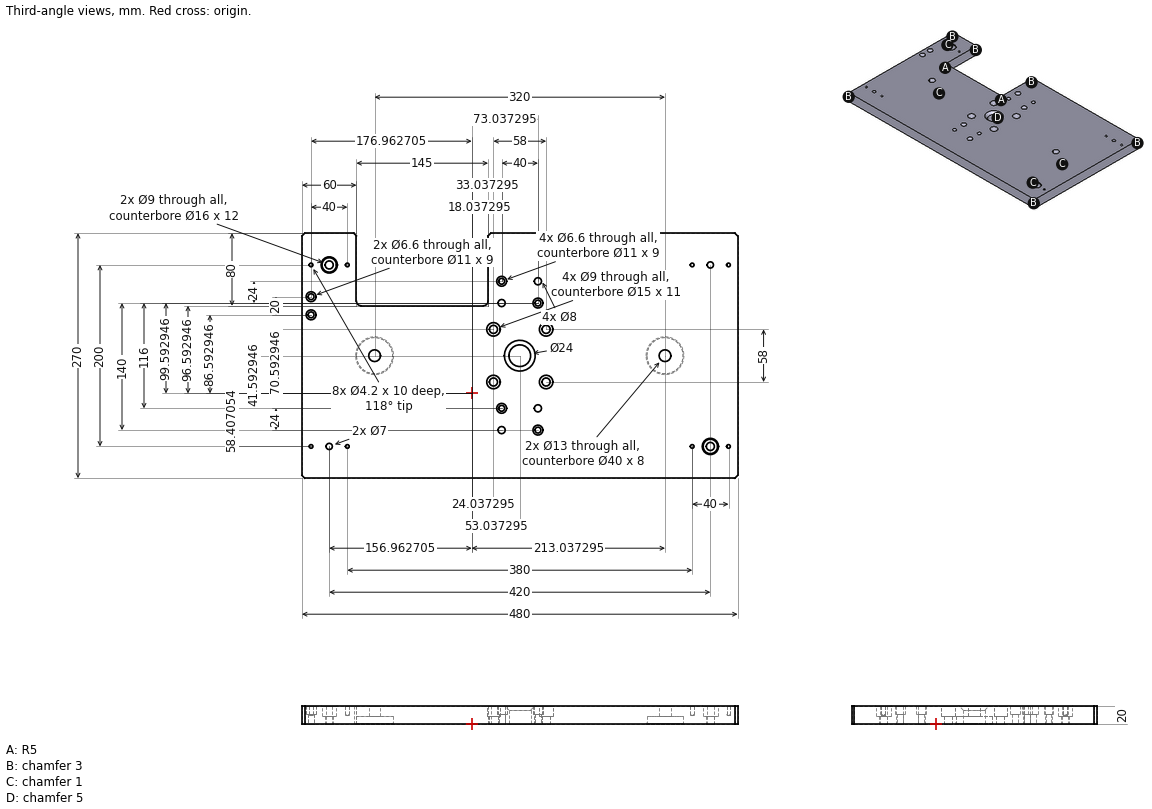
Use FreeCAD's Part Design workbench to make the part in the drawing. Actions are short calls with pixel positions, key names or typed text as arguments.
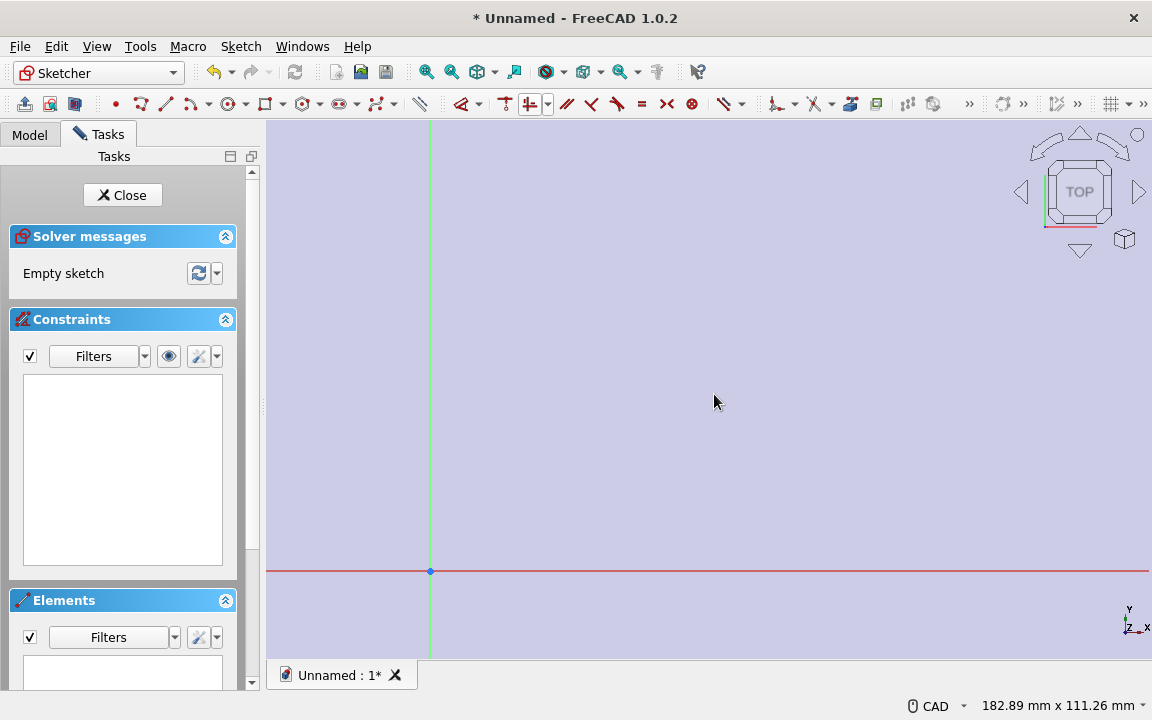
key(g)
key(c)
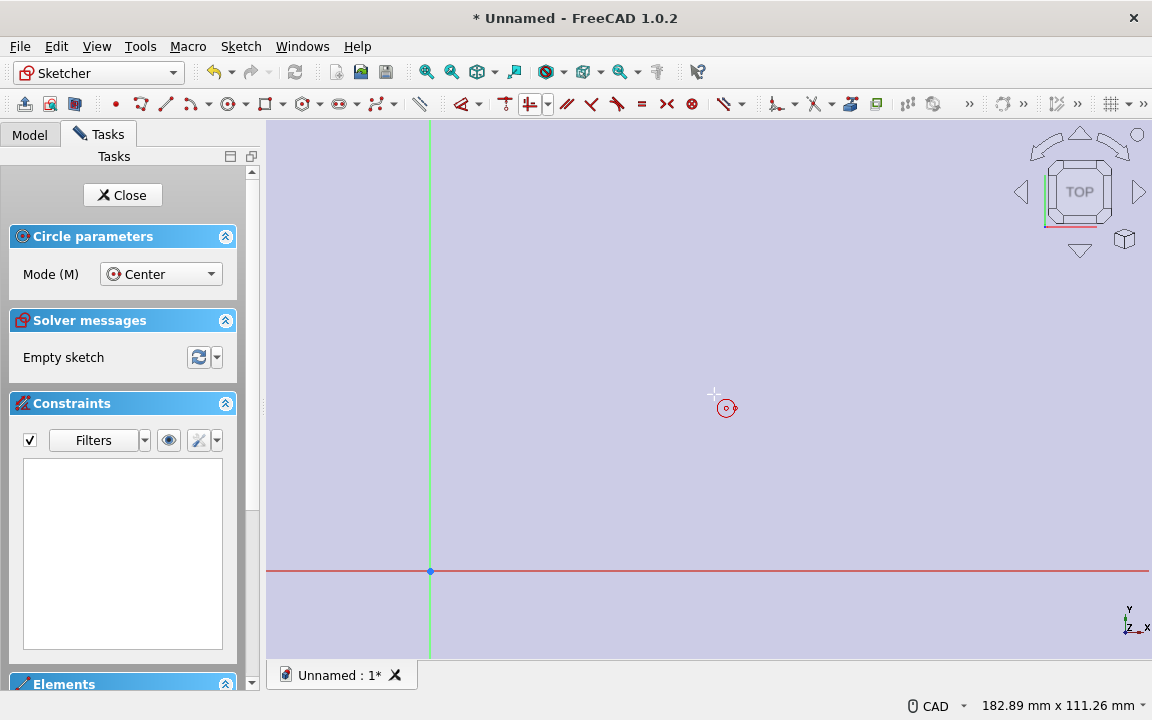
click(547, 229)
click(562, 214)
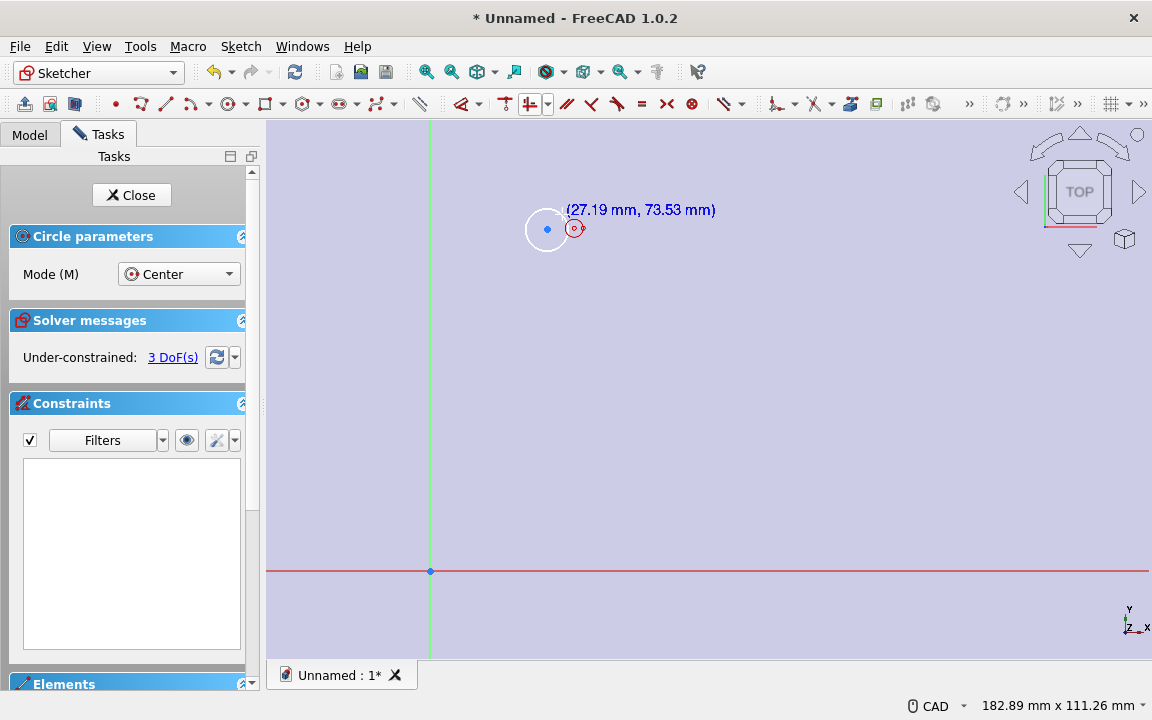
click(828, 229)
click(843, 214)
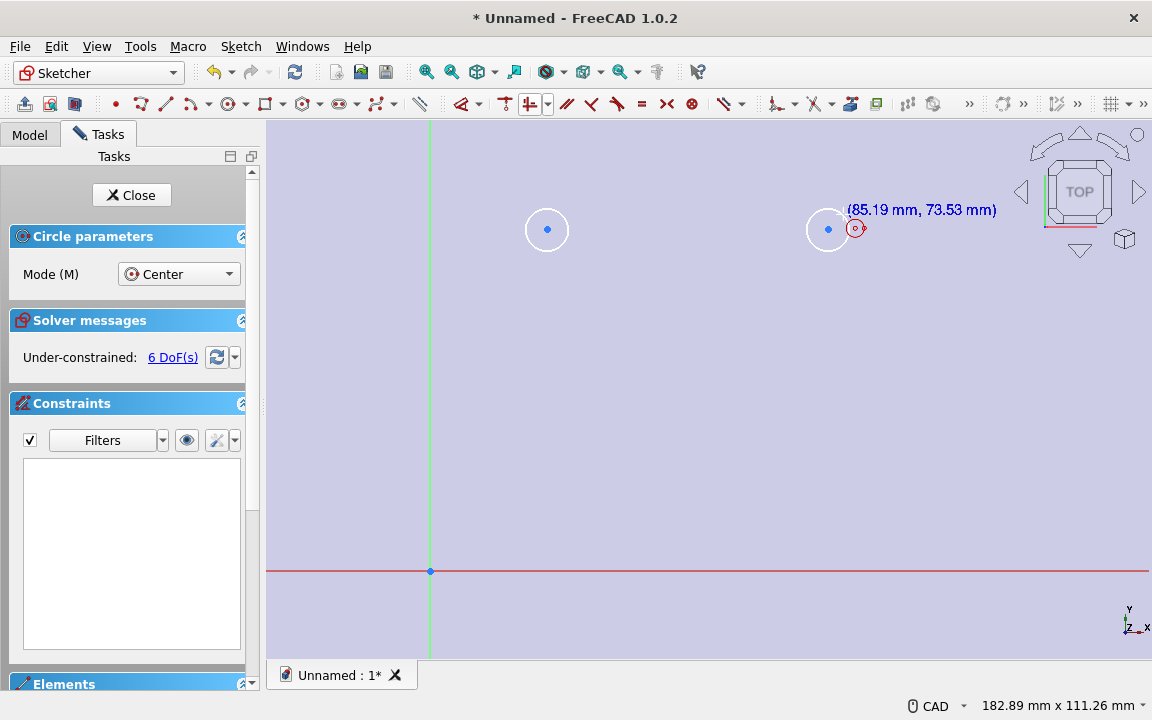
click(828, 510)
click(843, 495)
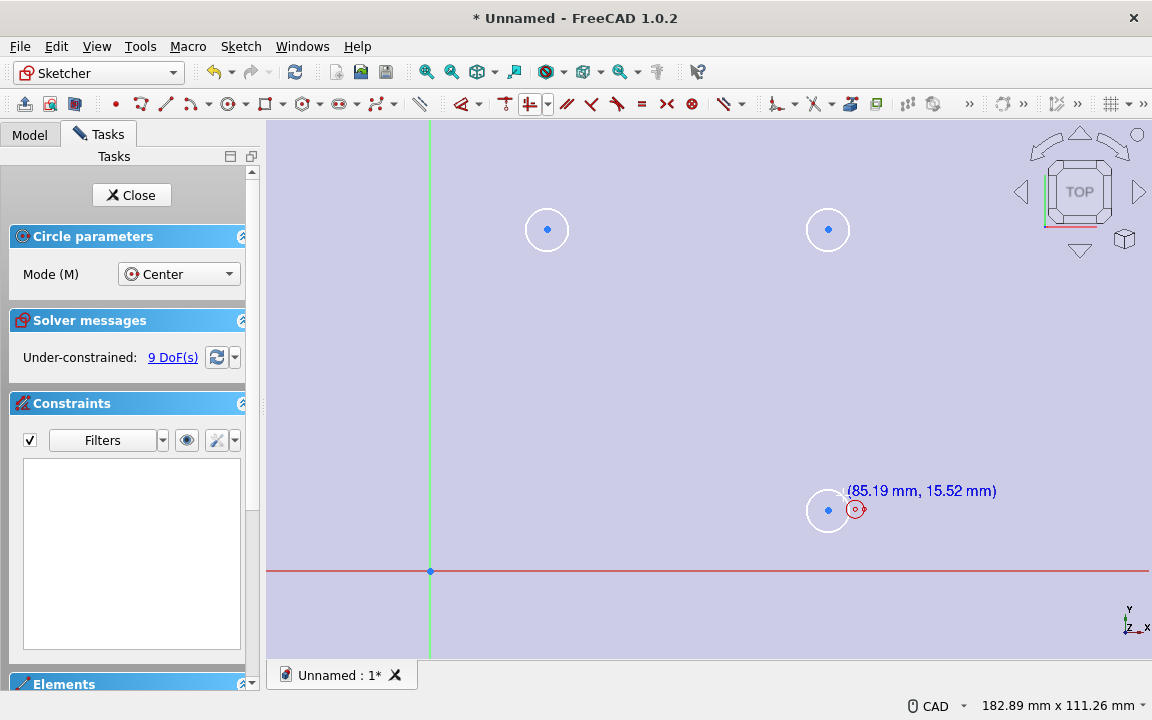
click(547, 510)
click(562, 495)
key(Escape)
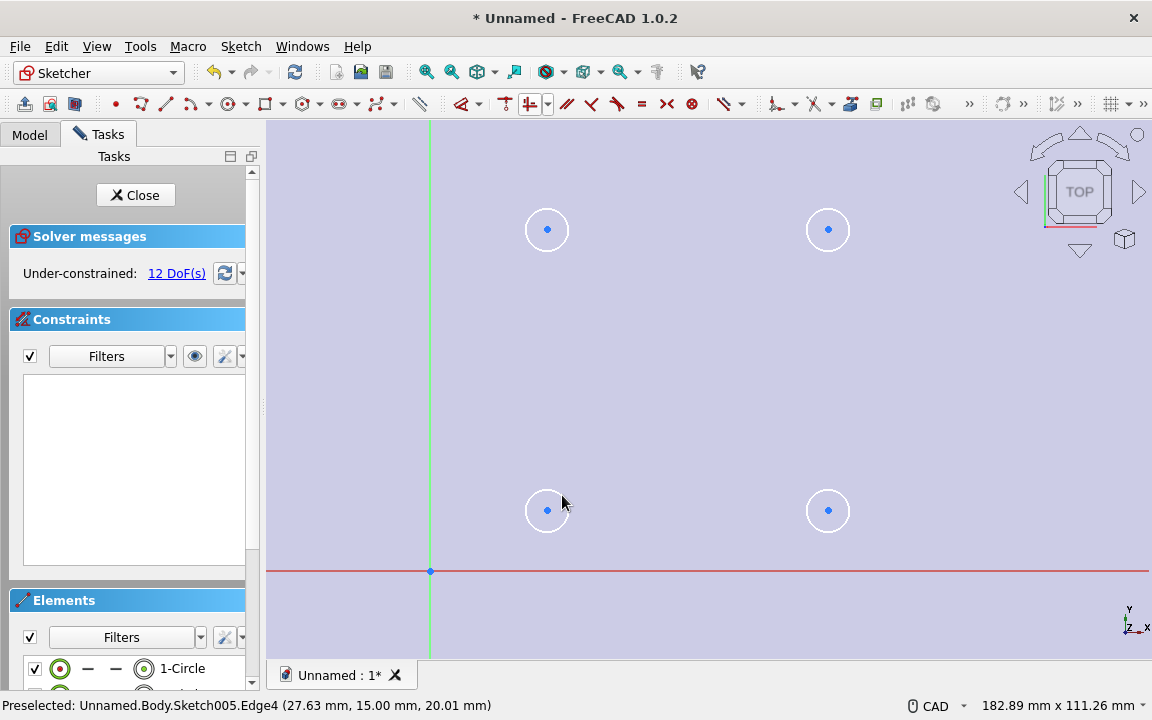
click(562, 215)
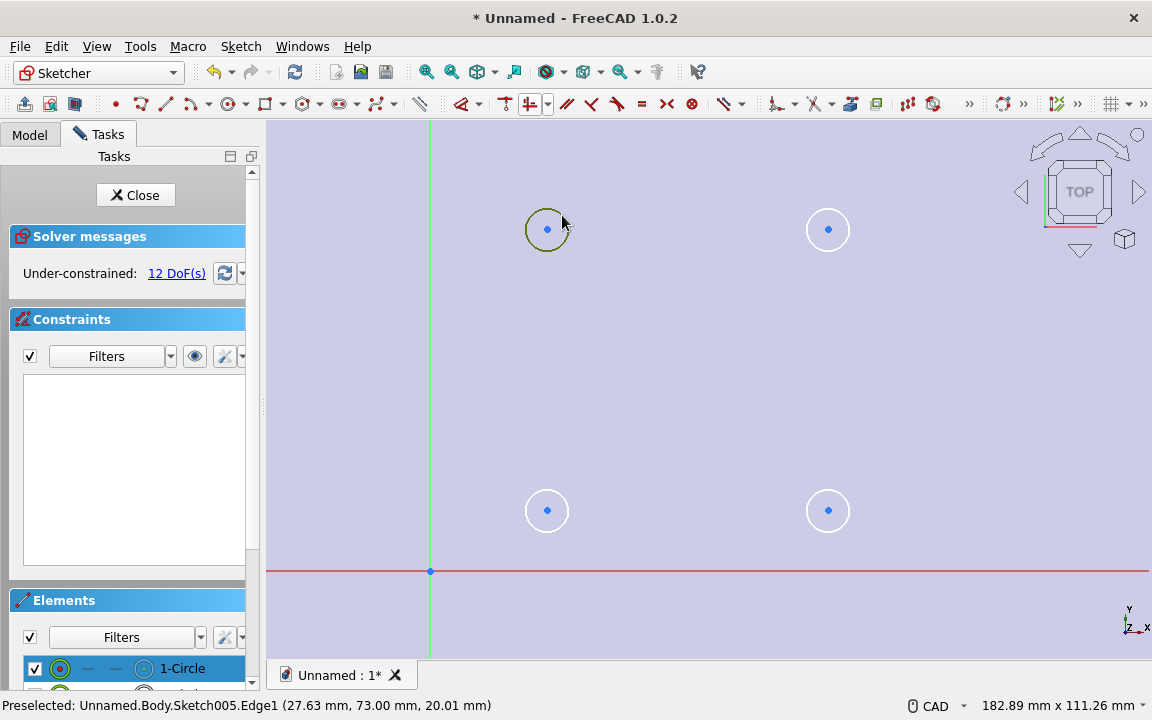
click(843, 215)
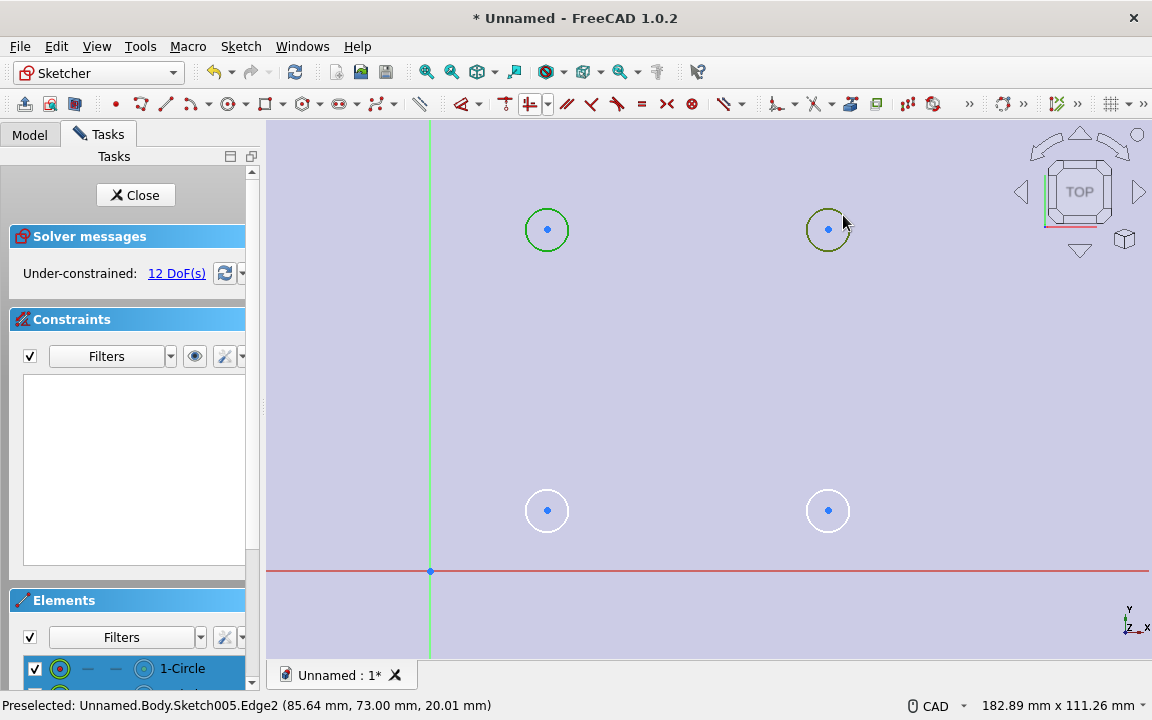
click(843, 496)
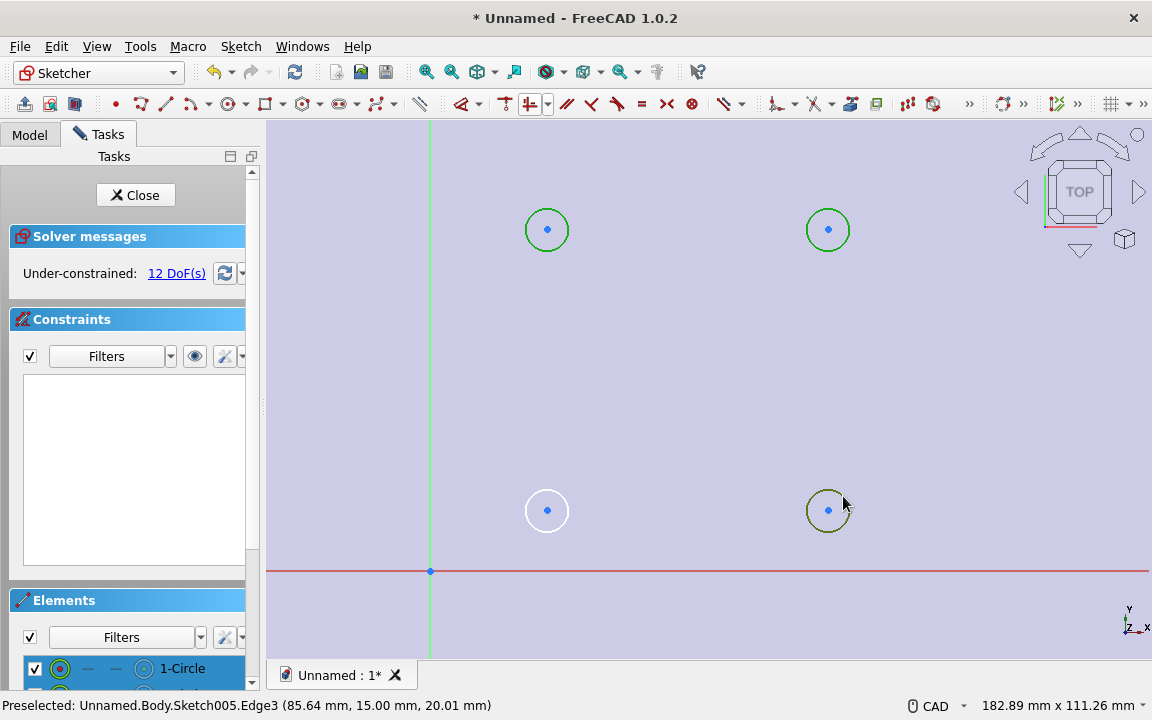
click(562, 496)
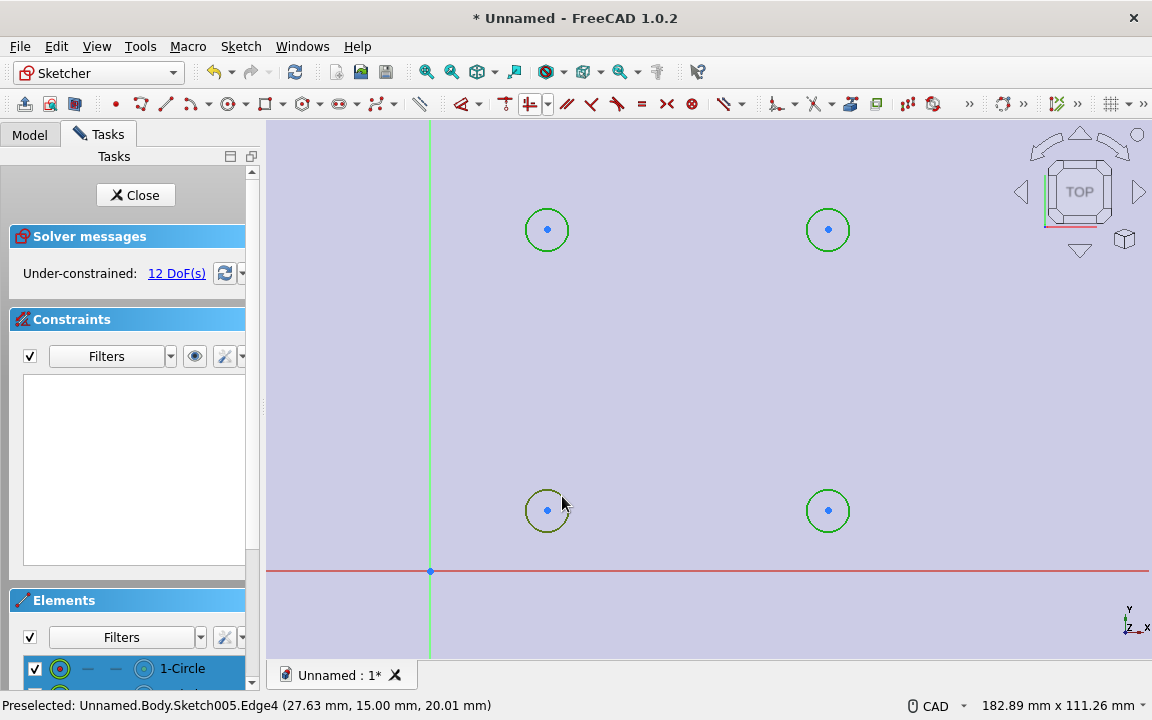
key(e)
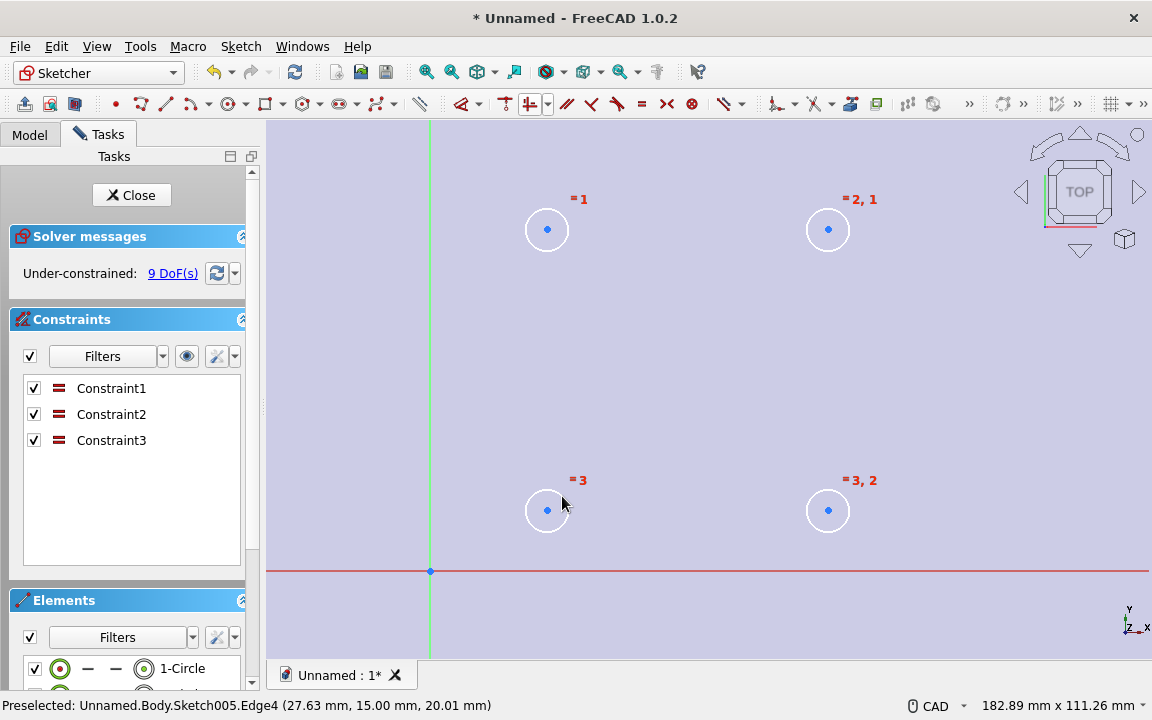
click(547, 230)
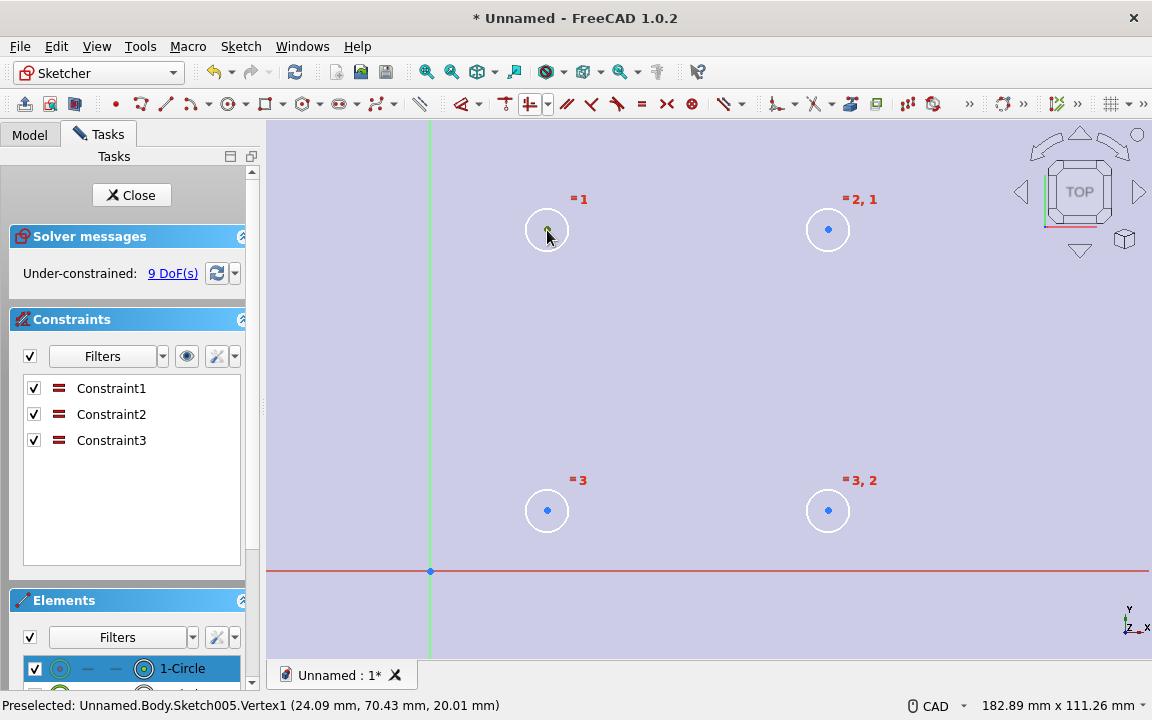
click(828, 230)